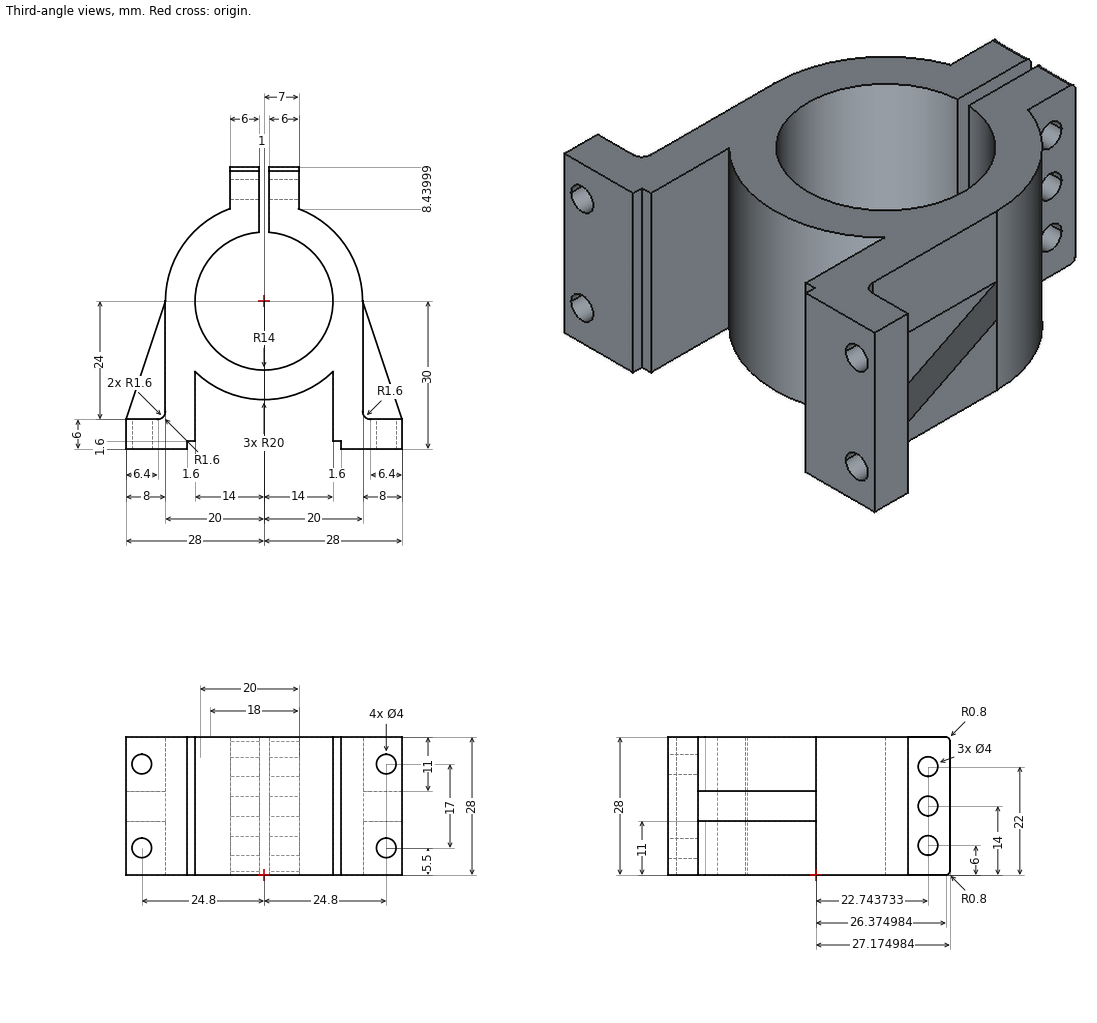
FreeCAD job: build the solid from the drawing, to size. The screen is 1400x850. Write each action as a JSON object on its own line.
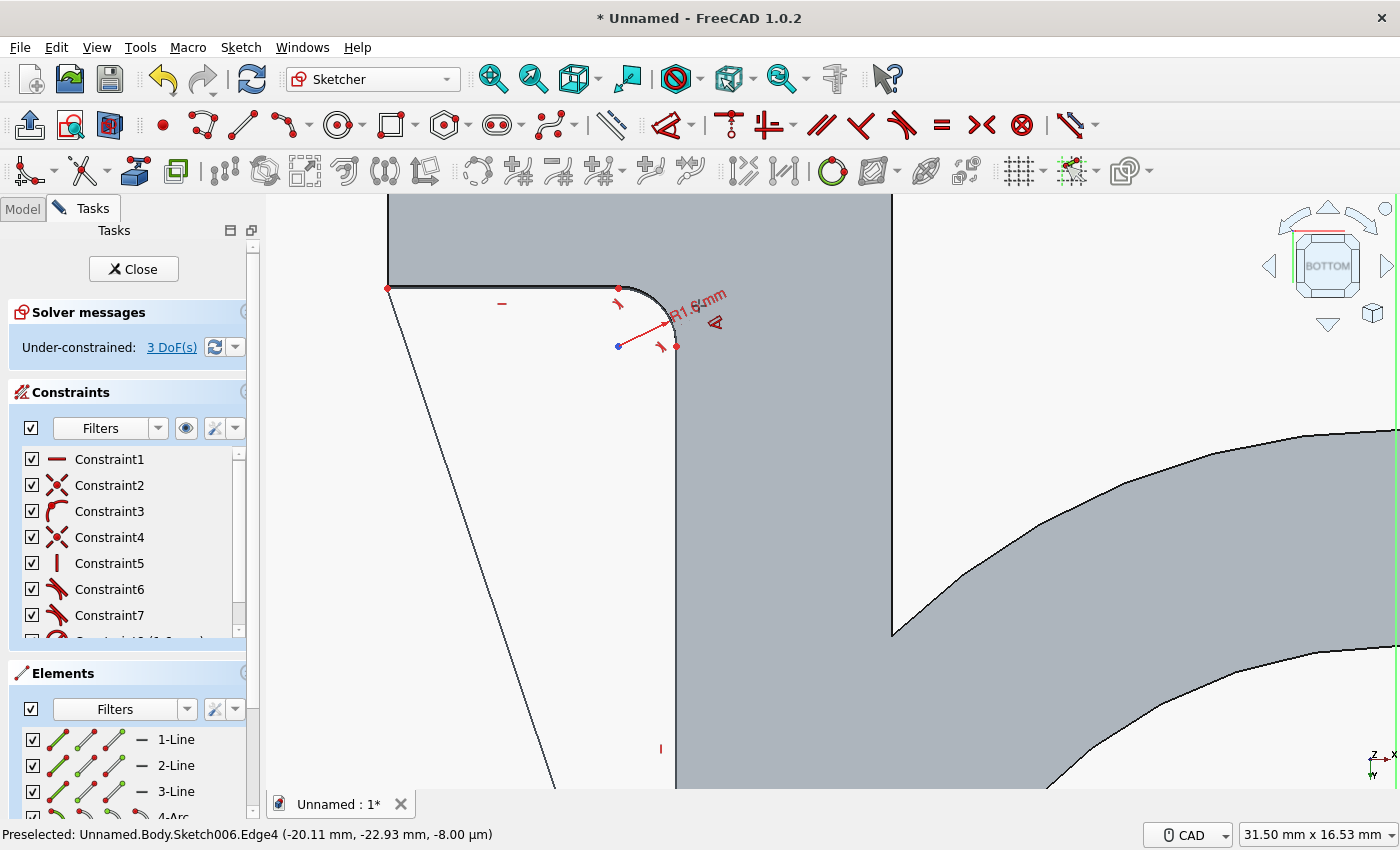
{"action": "left_click", "coordinate": [474, 547]}
{"action": "left_click", "coordinate": [532, 254]}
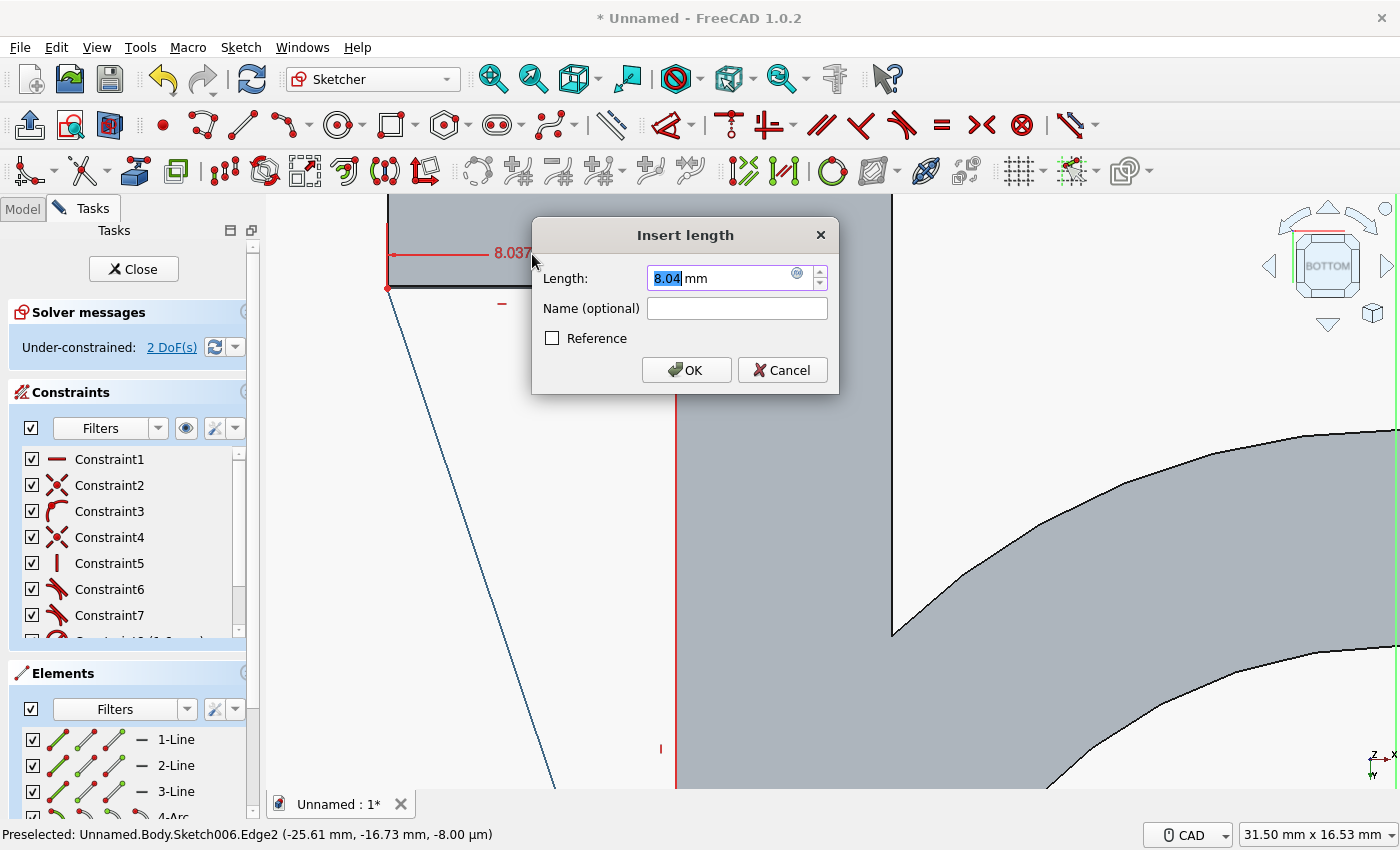
{"action": "type", "text": "8"}
{"action": "key", "text": "Return"}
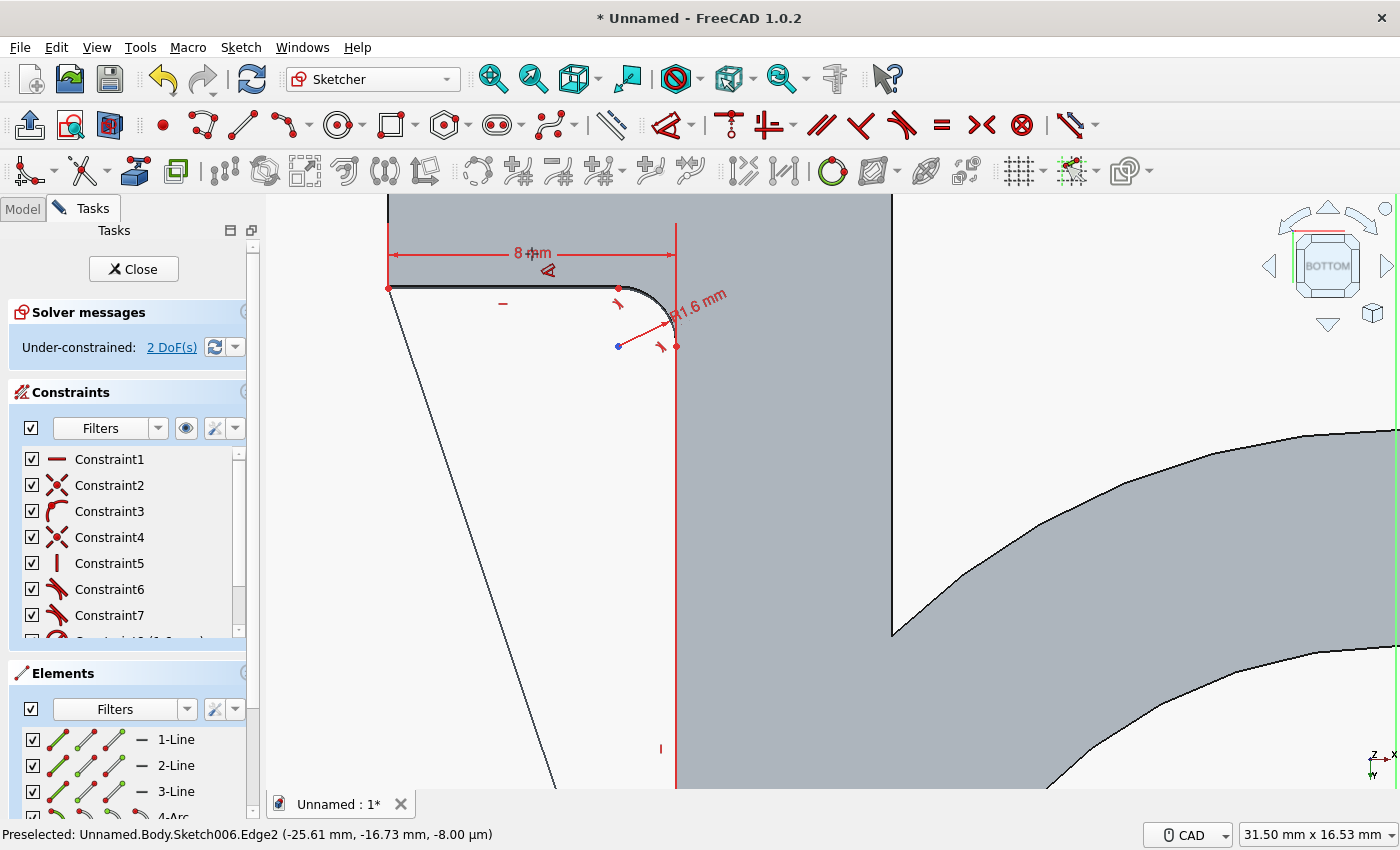
{"action": "left_click", "coordinate": [619, 288]}
{"action": "left_click", "coordinate": [585, 525]}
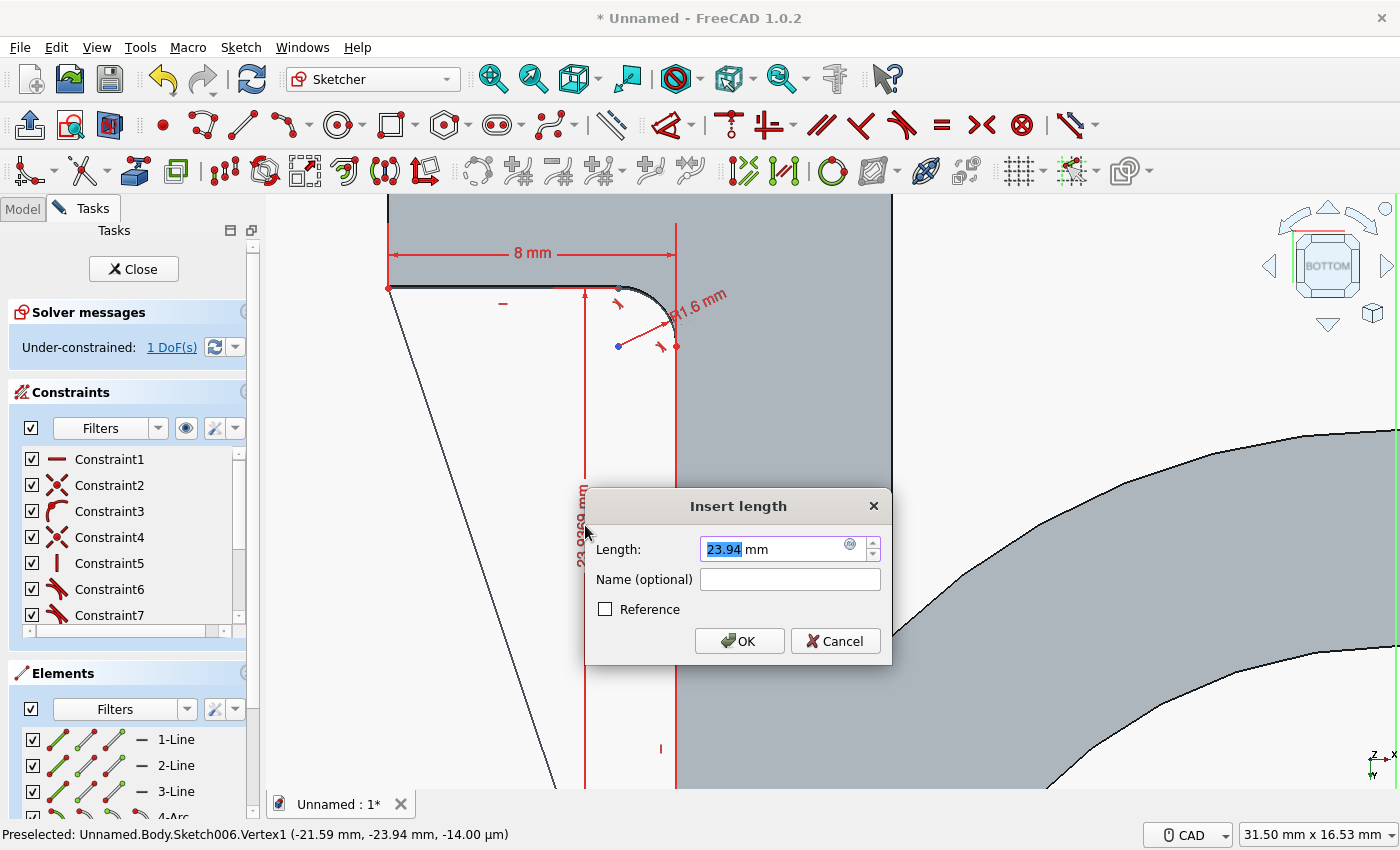
{"action": "type", "text": "24"}
{"action": "key", "text": "Return"}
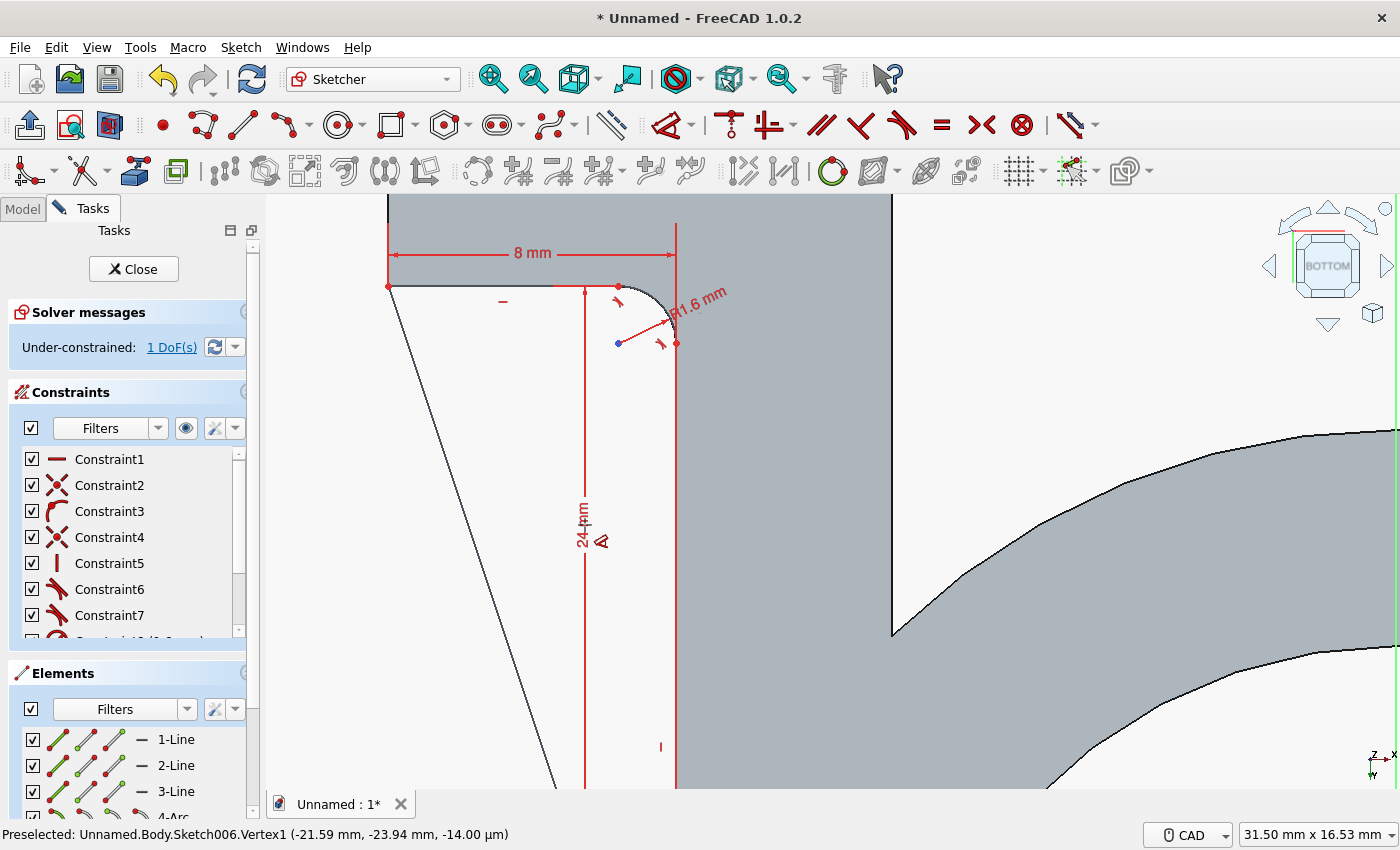
{"action": "left_click", "coordinate": [388, 286]}
{"action": "left_click", "coordinate": [812, 252]}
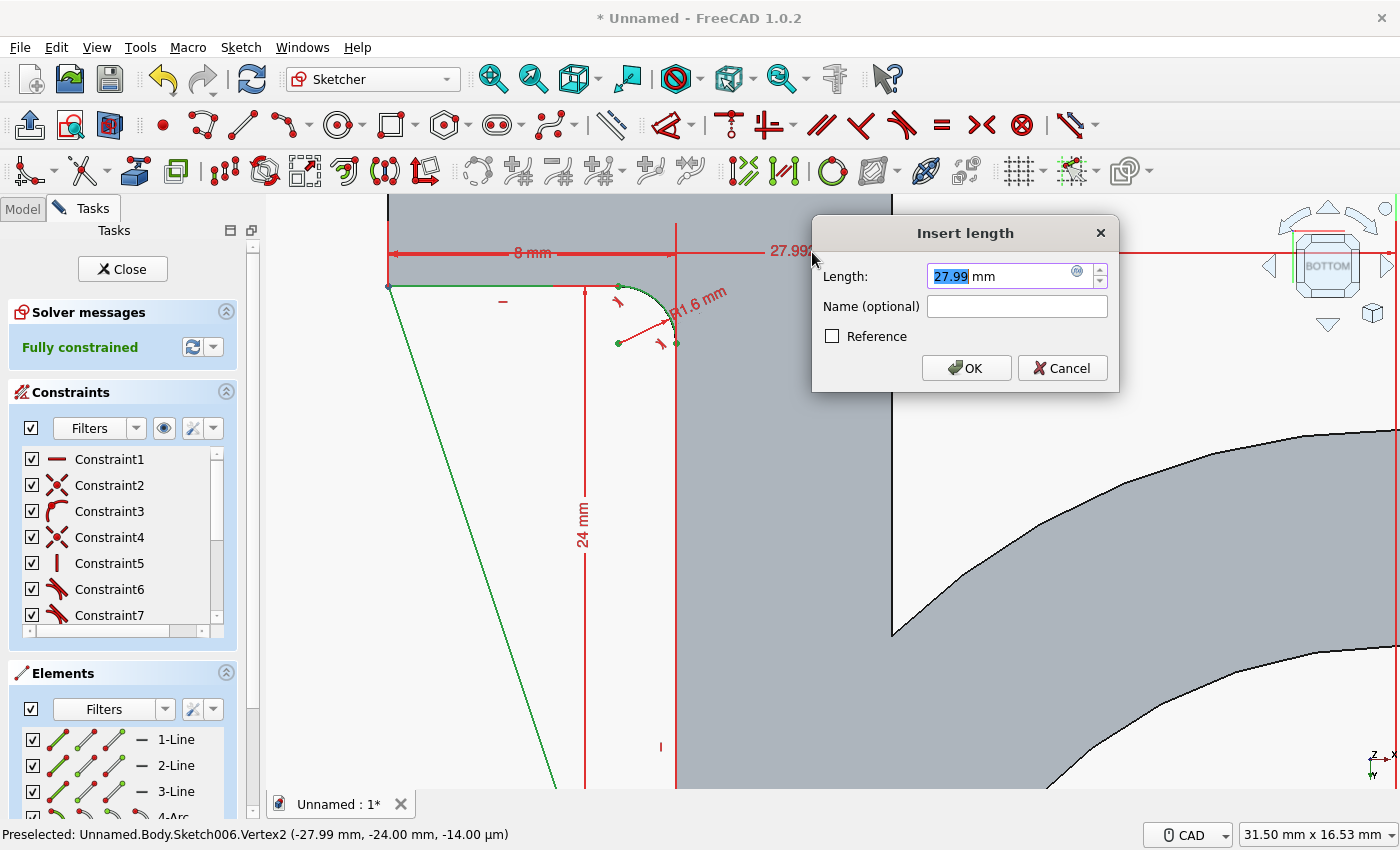
{"action": "type", "text": "28"}
{"action": "key", "text": "Return"}
{"action": "key", "text": "Escape"}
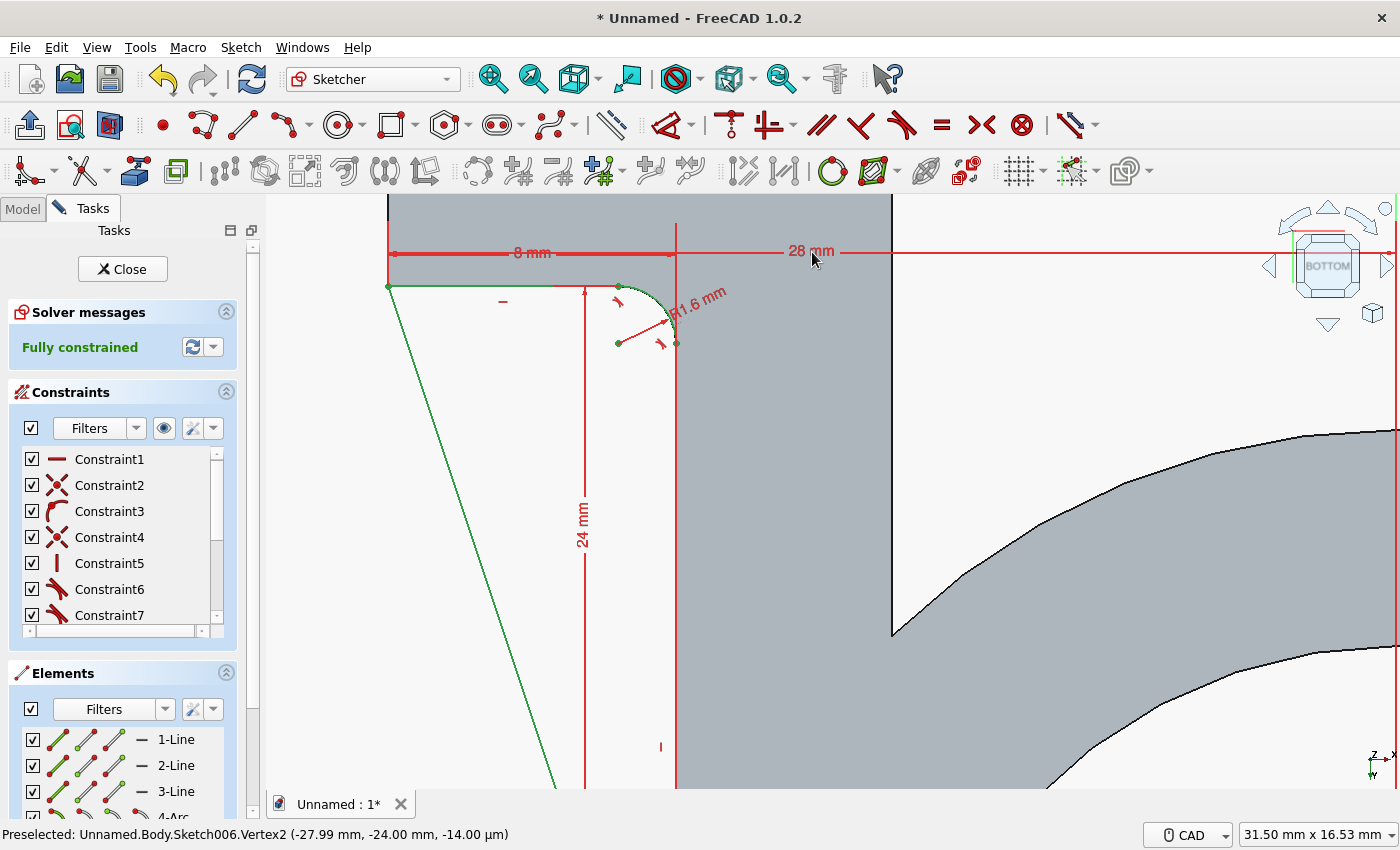
{"action": "left_click", "coordinate": [123, 269]}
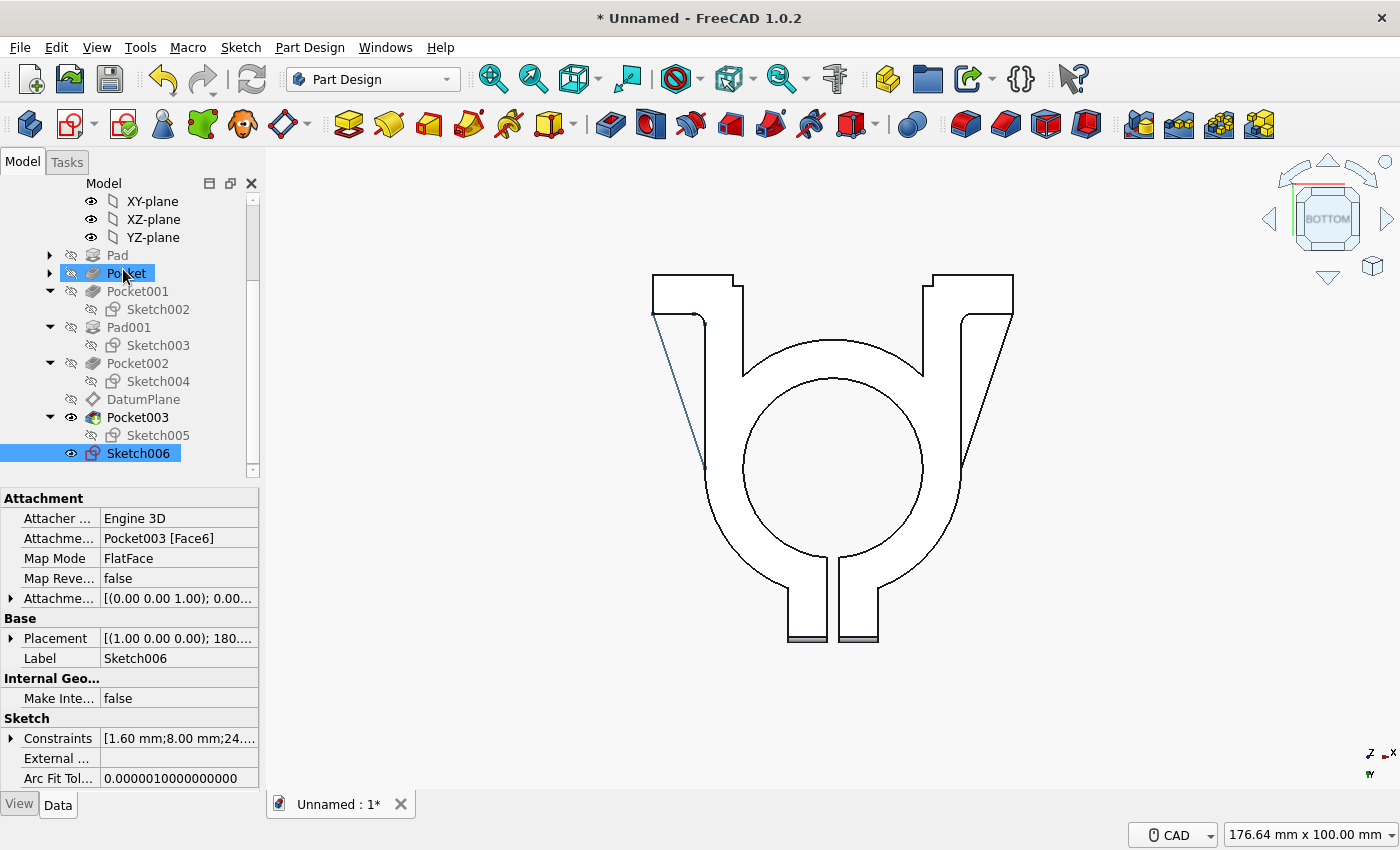
{"action": "left_click", "coordinate": [350, 124]}